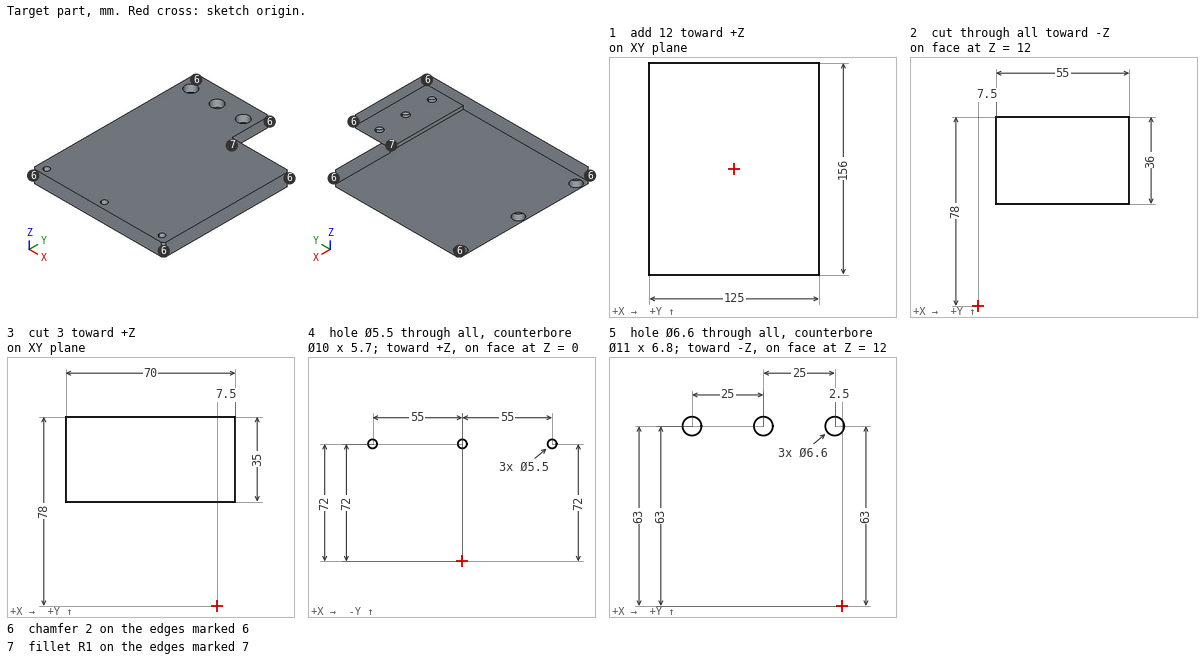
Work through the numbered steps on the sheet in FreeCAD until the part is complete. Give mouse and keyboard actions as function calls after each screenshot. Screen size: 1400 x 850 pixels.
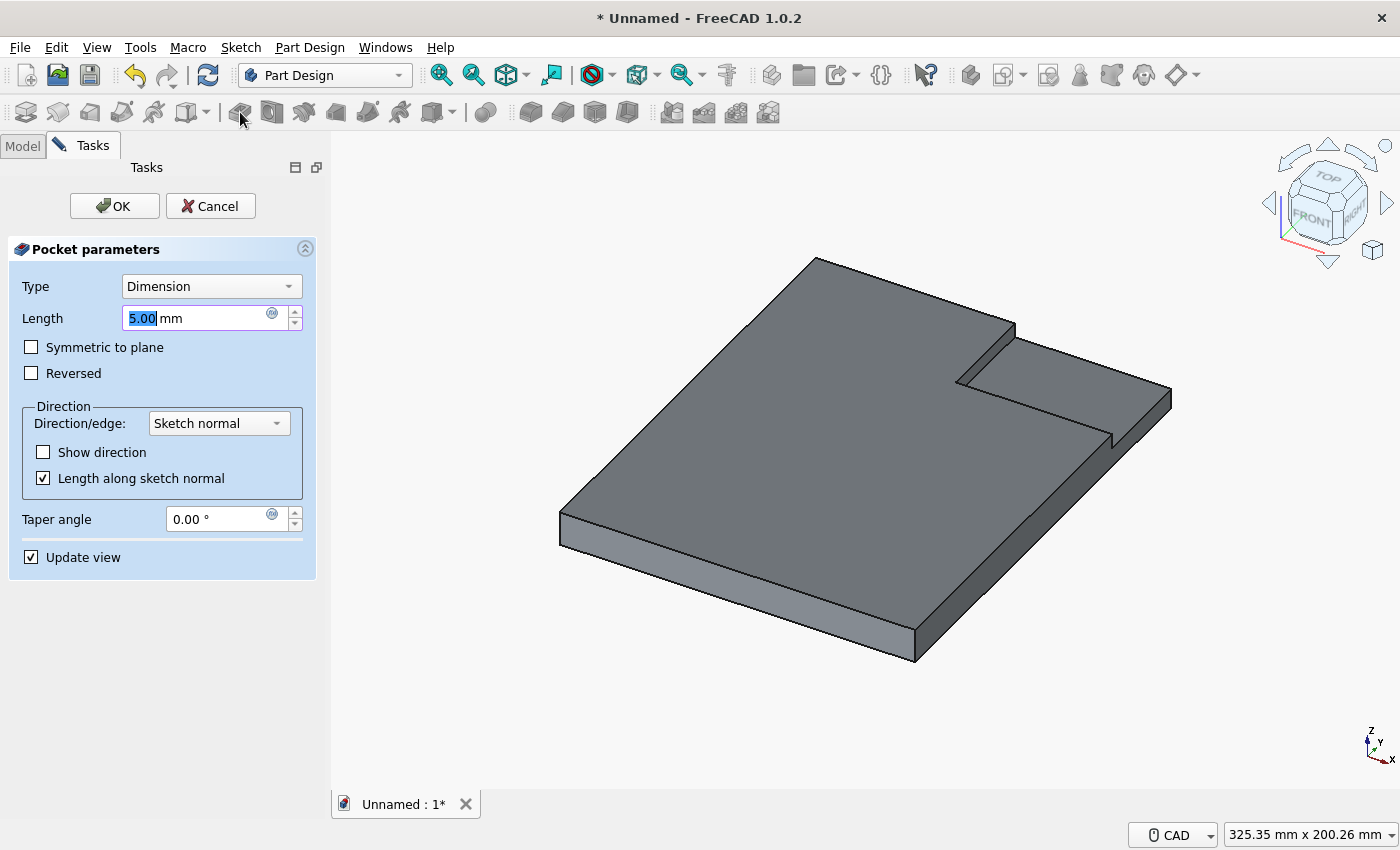
click(212, 286)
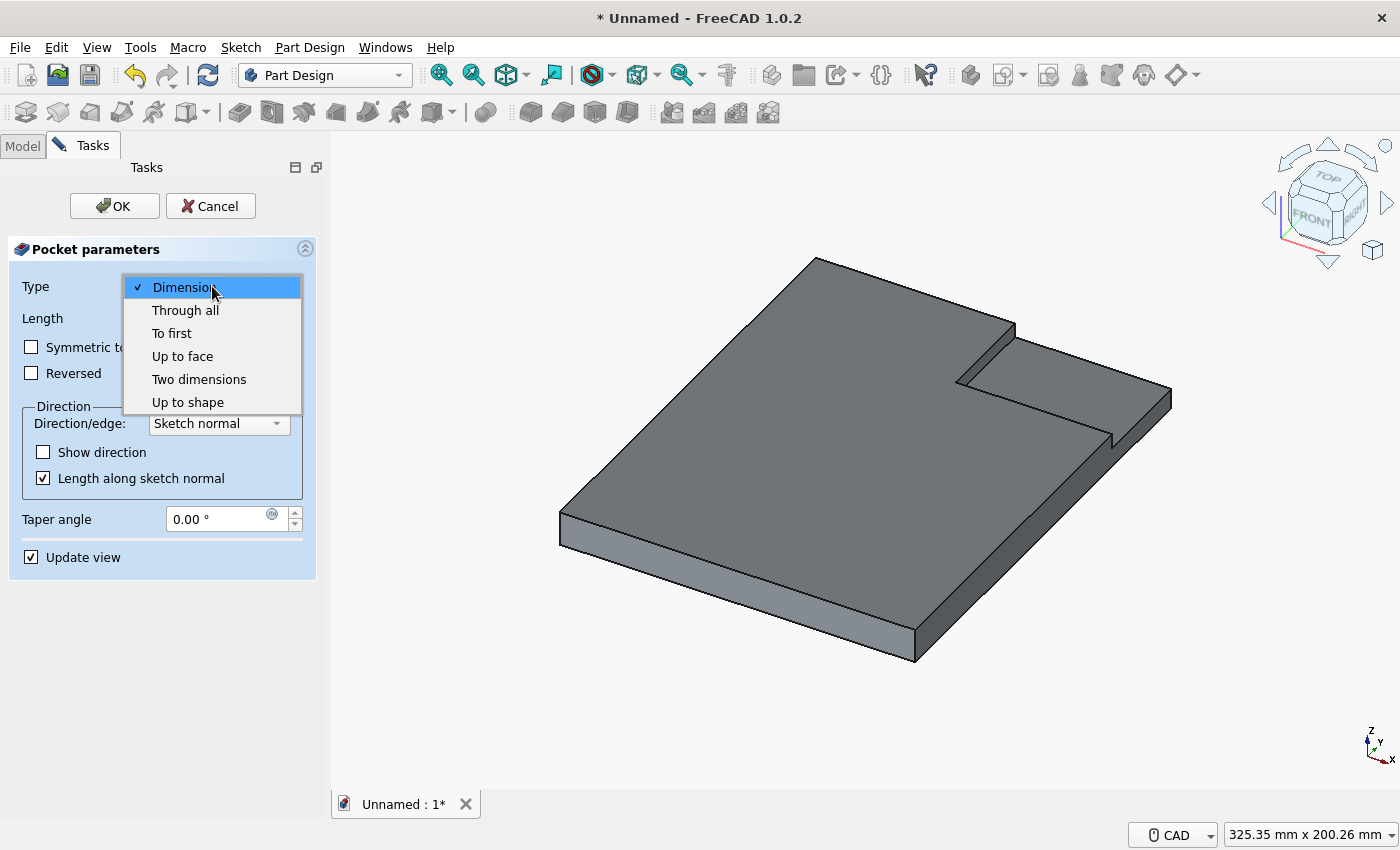
click(212, 310)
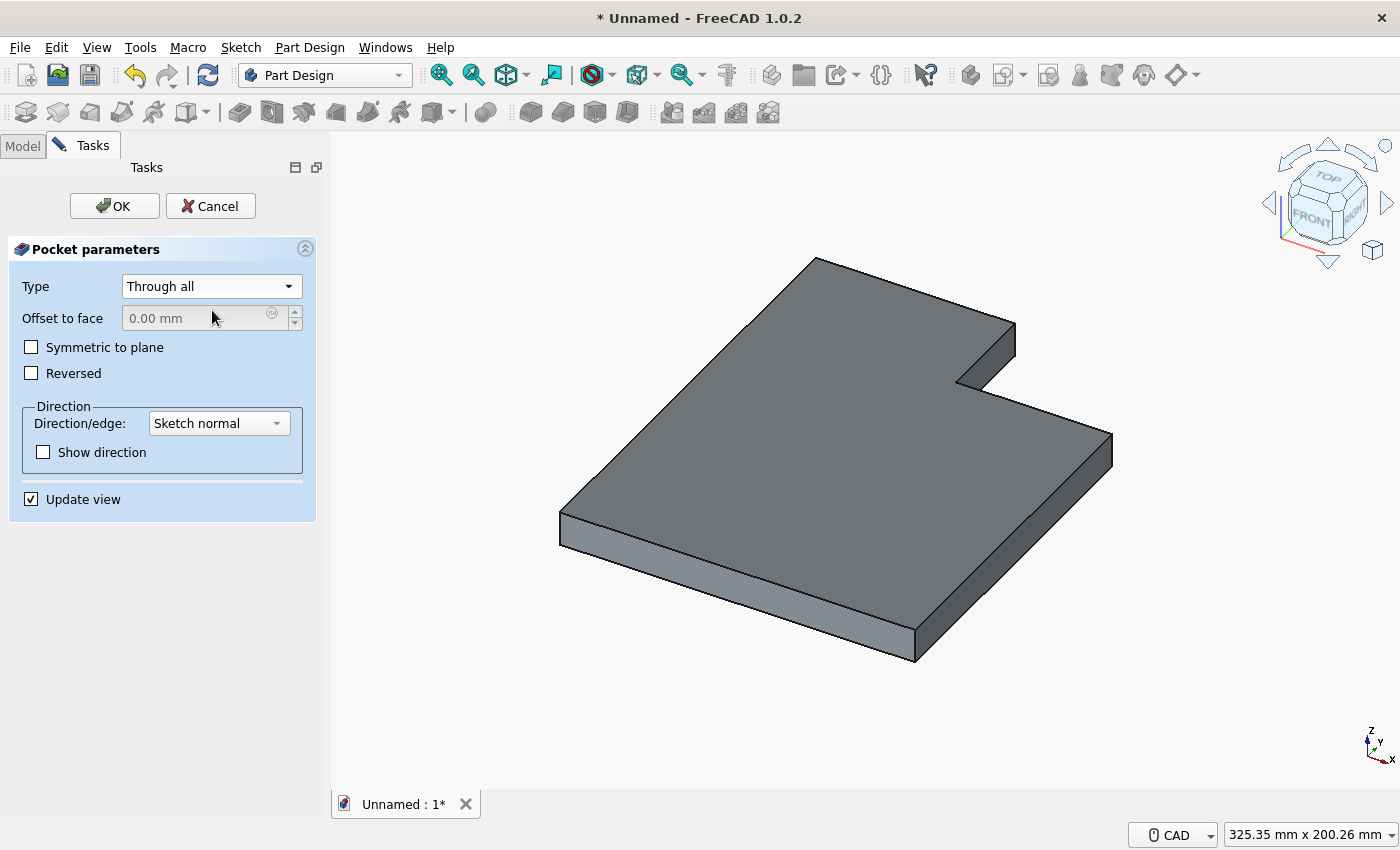
click(115, 206)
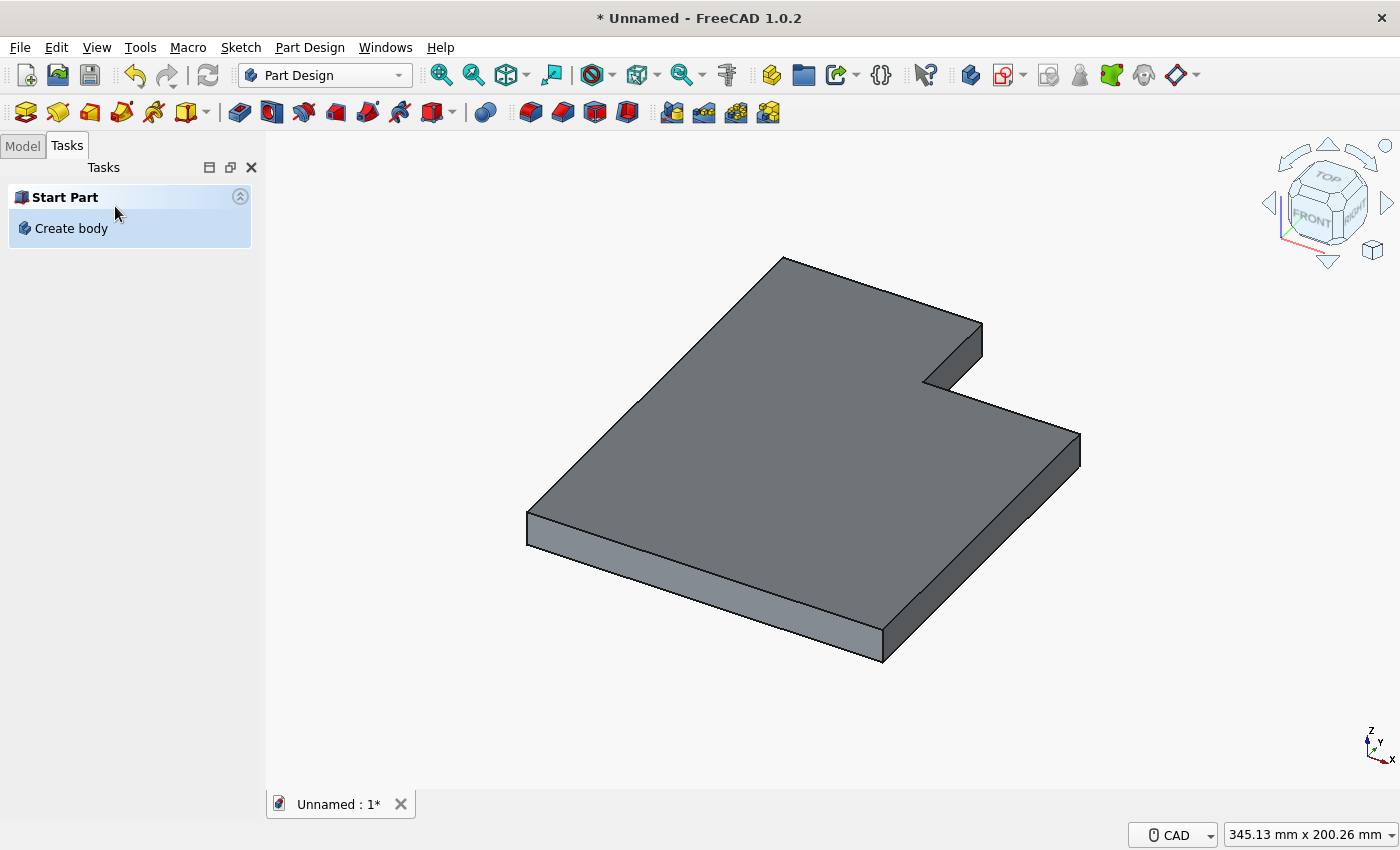
click(1004, 76)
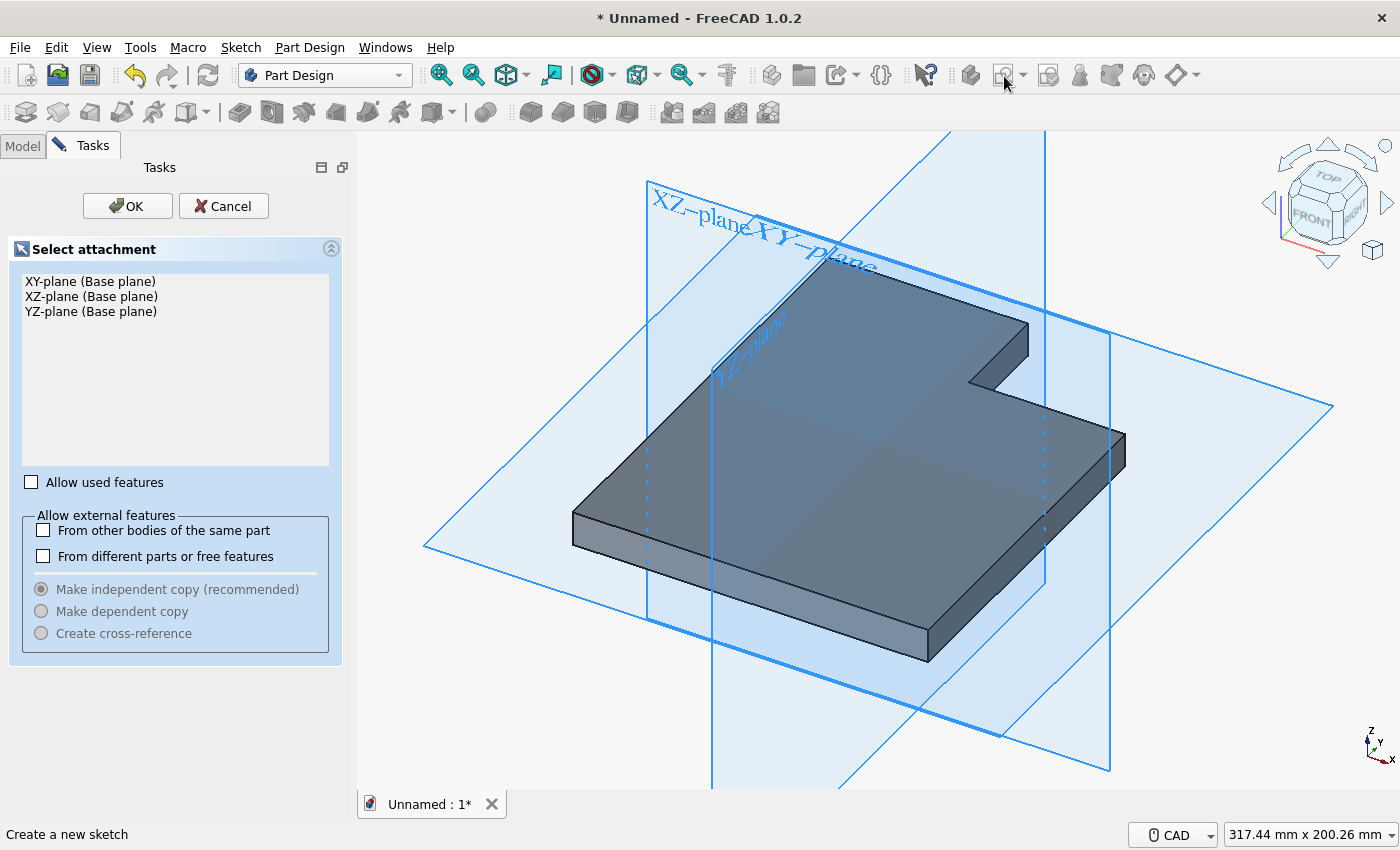
click(82, 282)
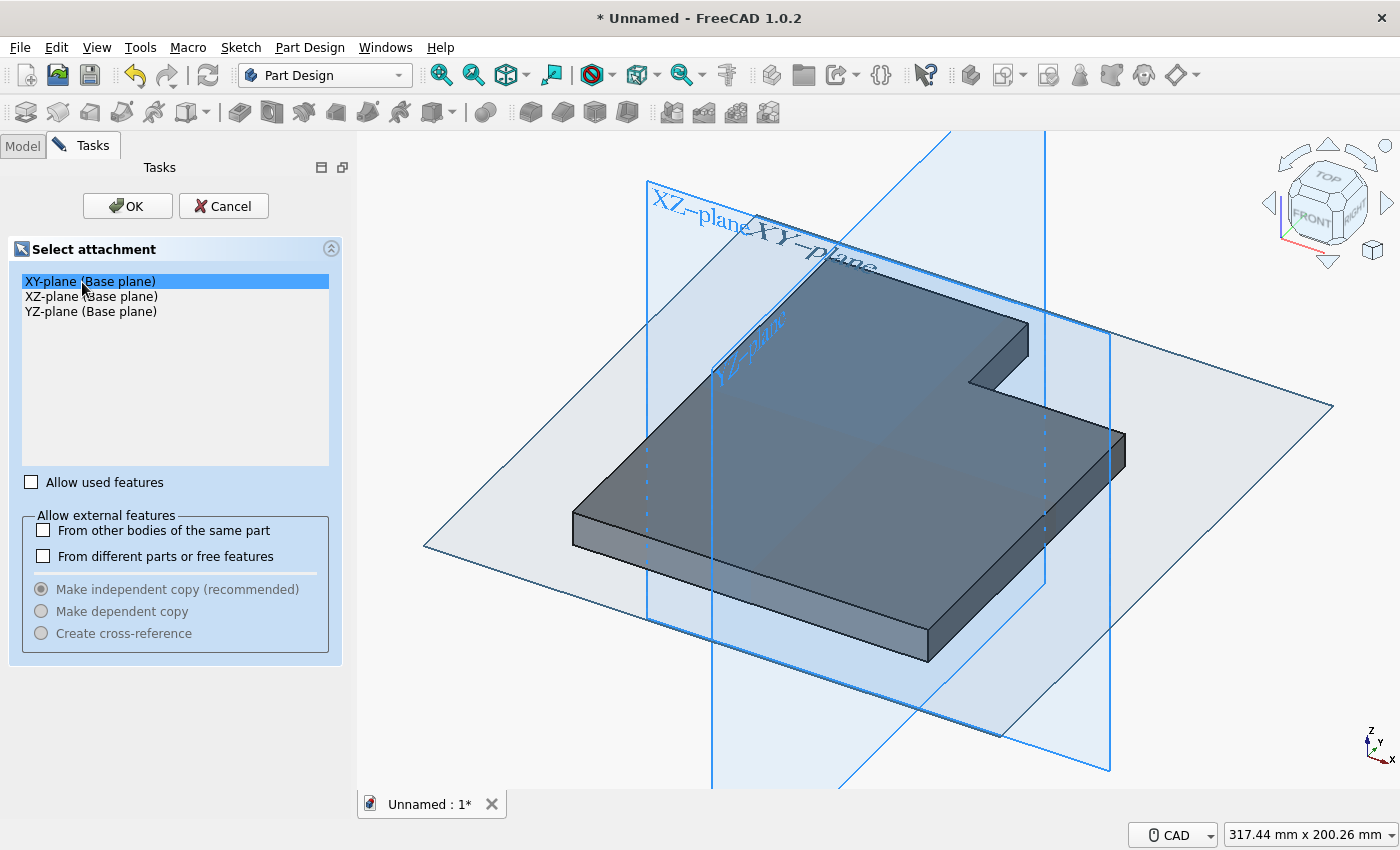
click(128, 206)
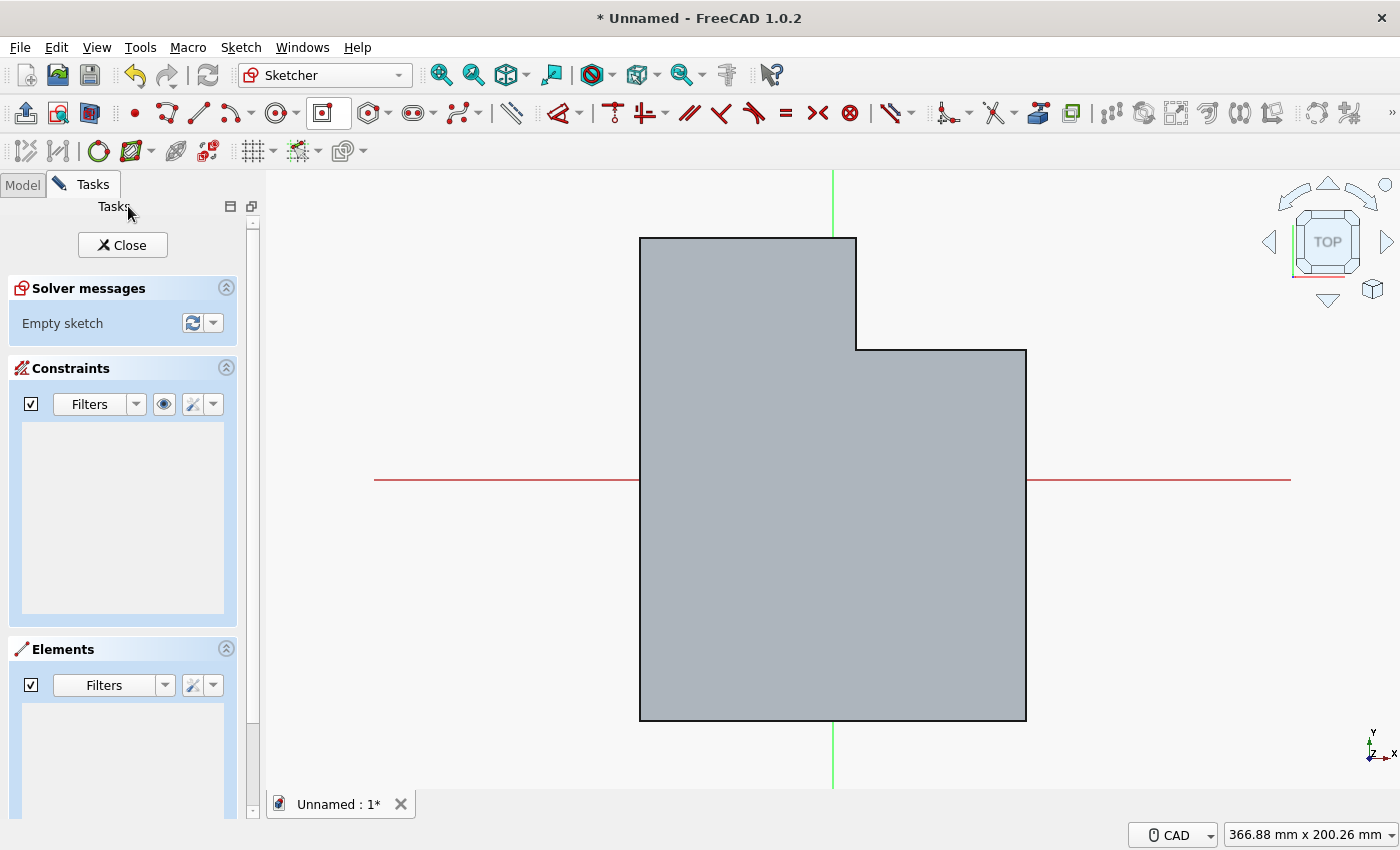
click(90, 114)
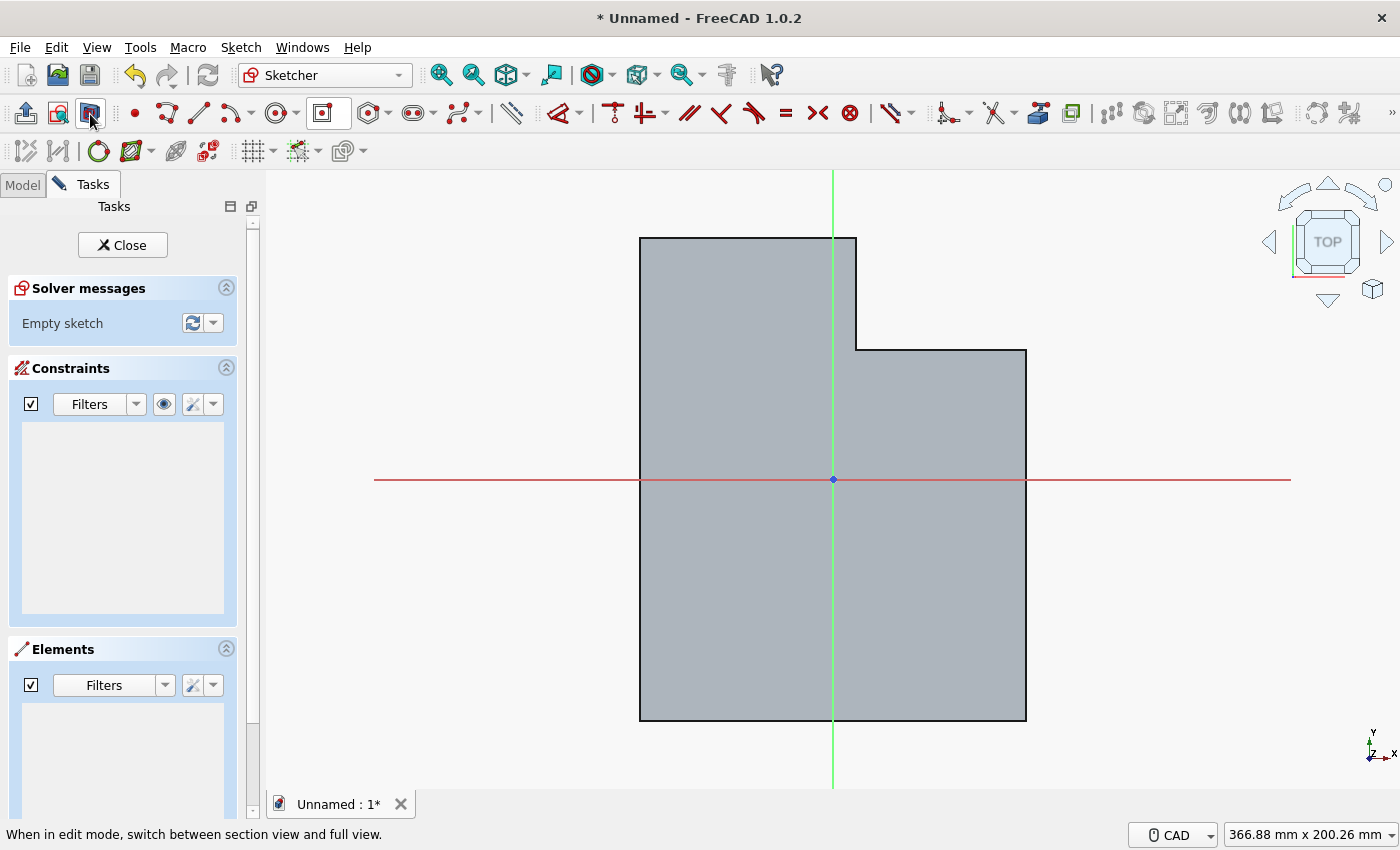
scroll(714, 198, up, 2)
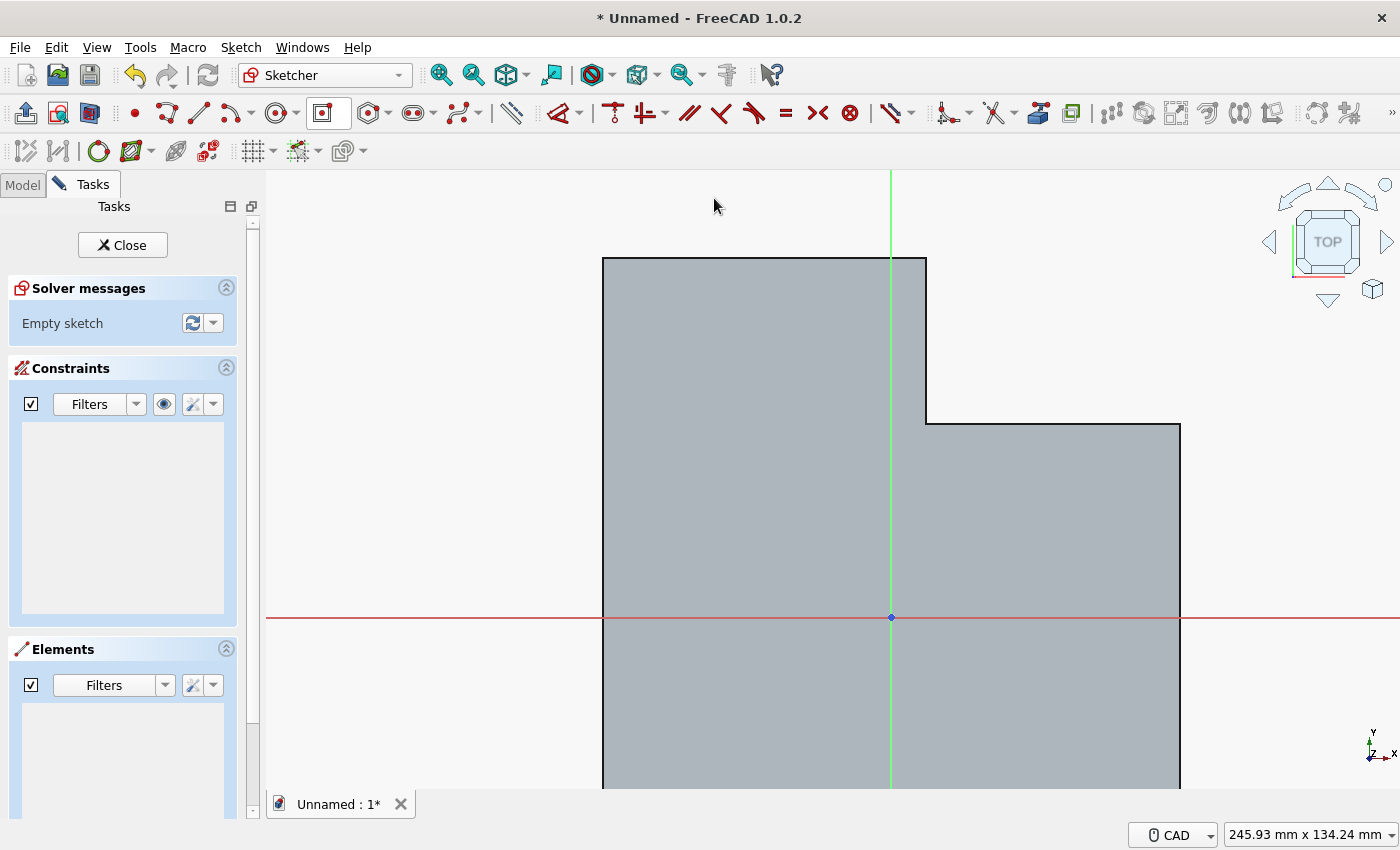
click(346, 114)